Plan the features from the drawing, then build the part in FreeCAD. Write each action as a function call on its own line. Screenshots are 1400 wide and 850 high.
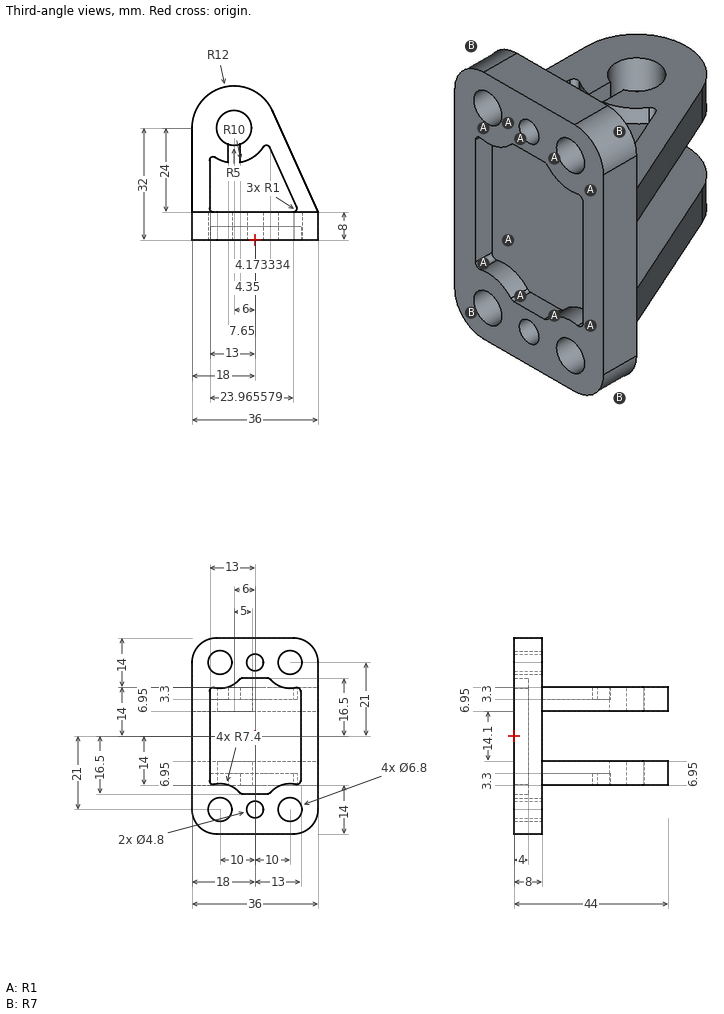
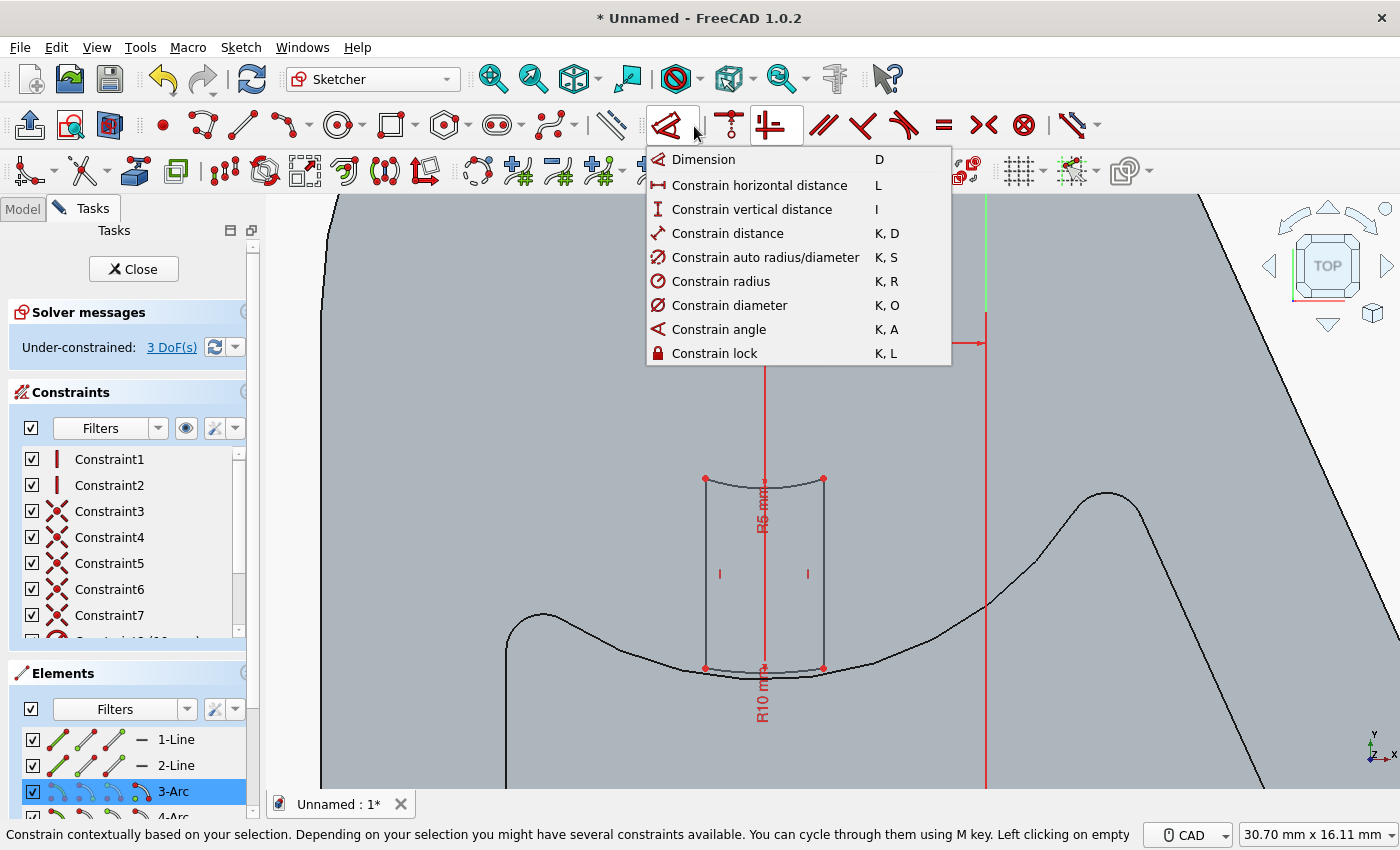
click(799, 209)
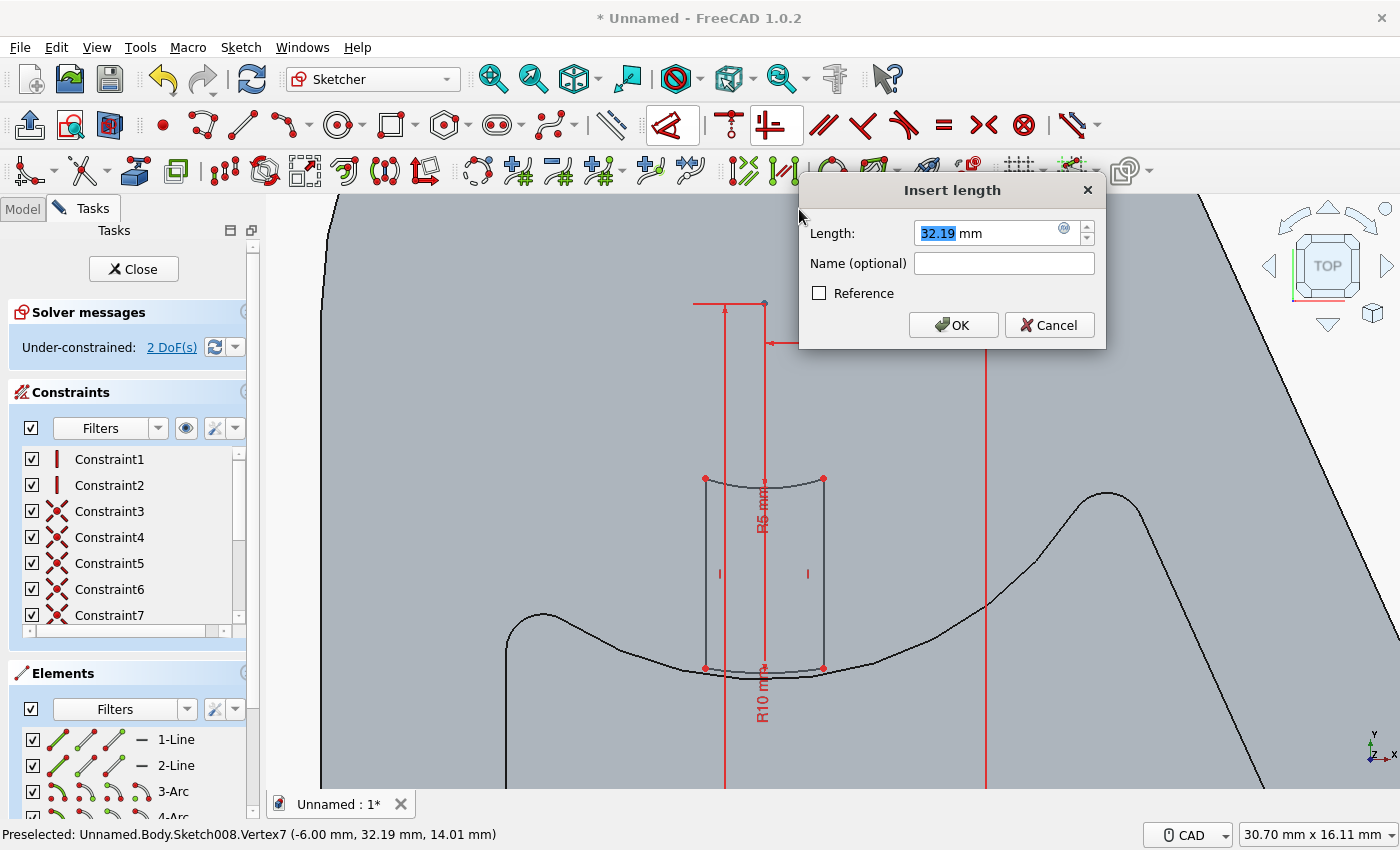
text(32)
key(Return)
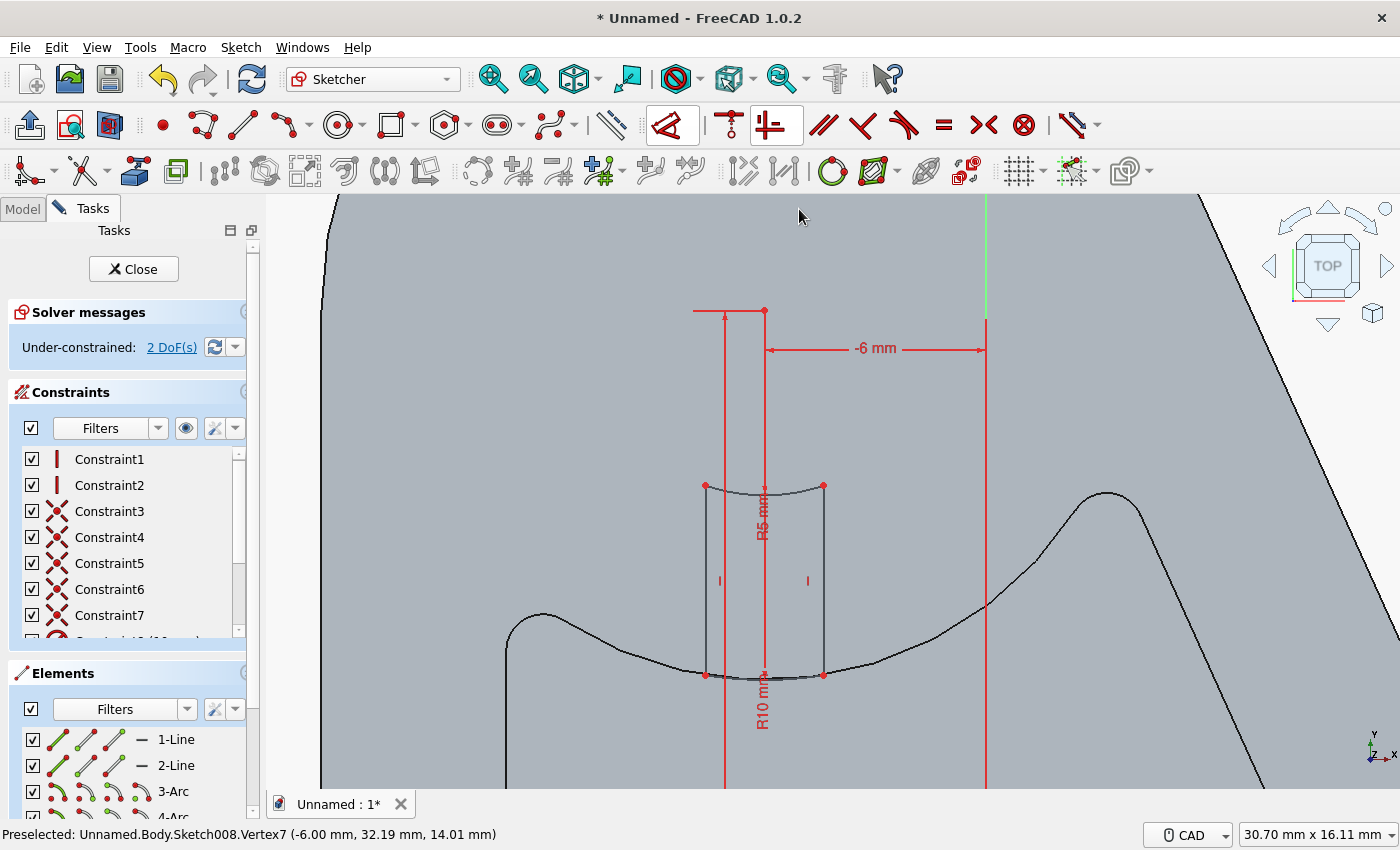
click(706, 486)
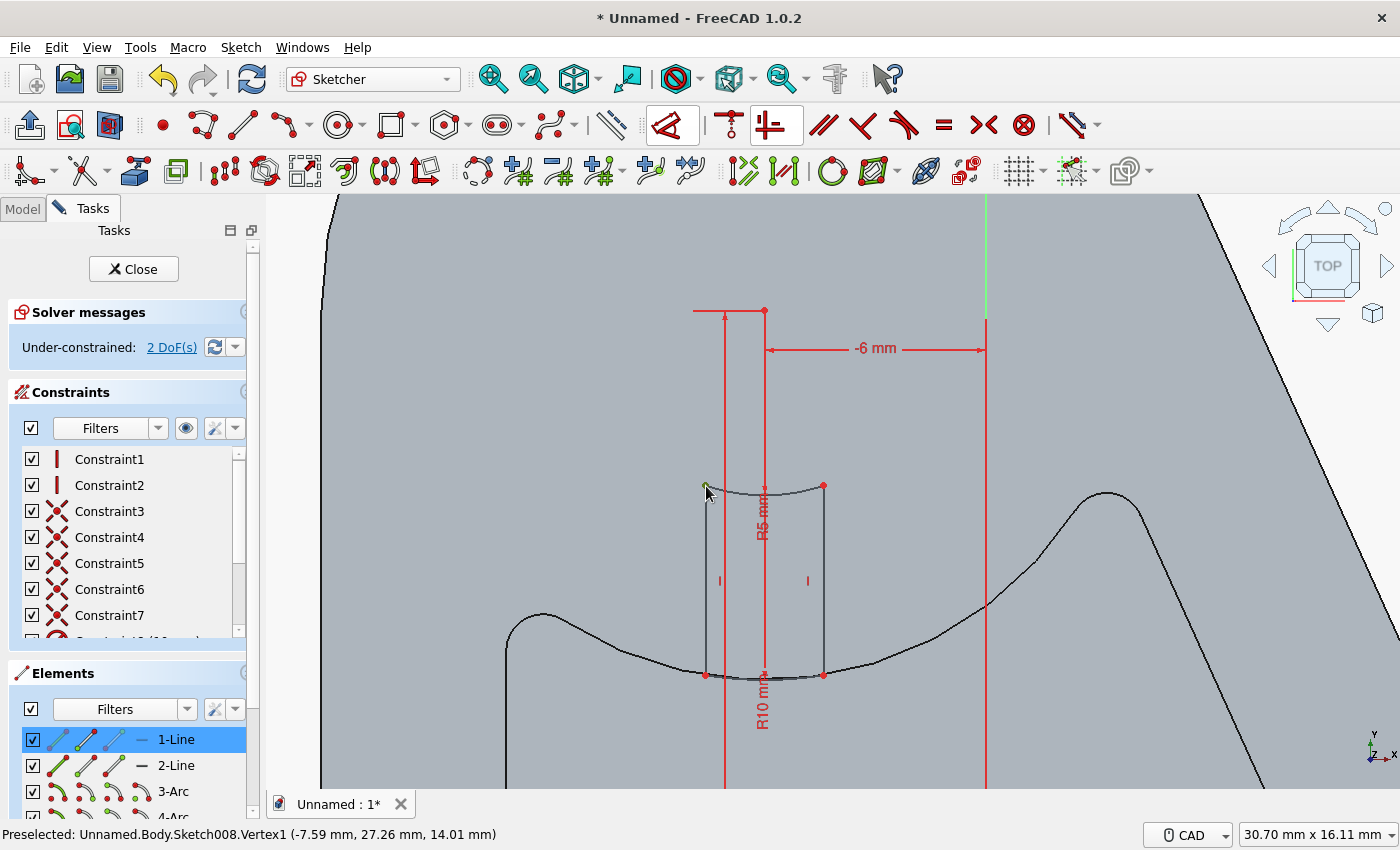
click(694, 126)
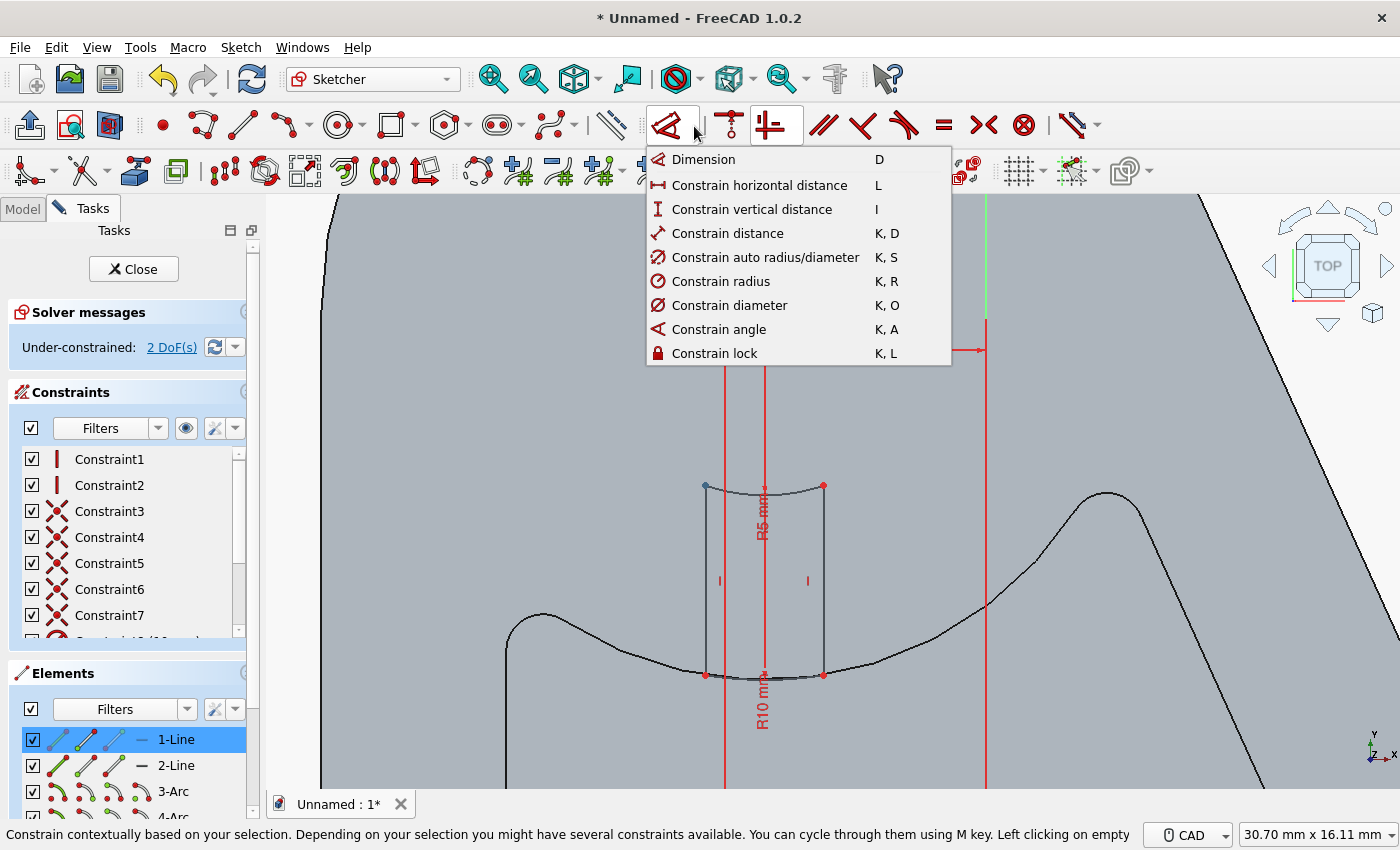
click(799, 185)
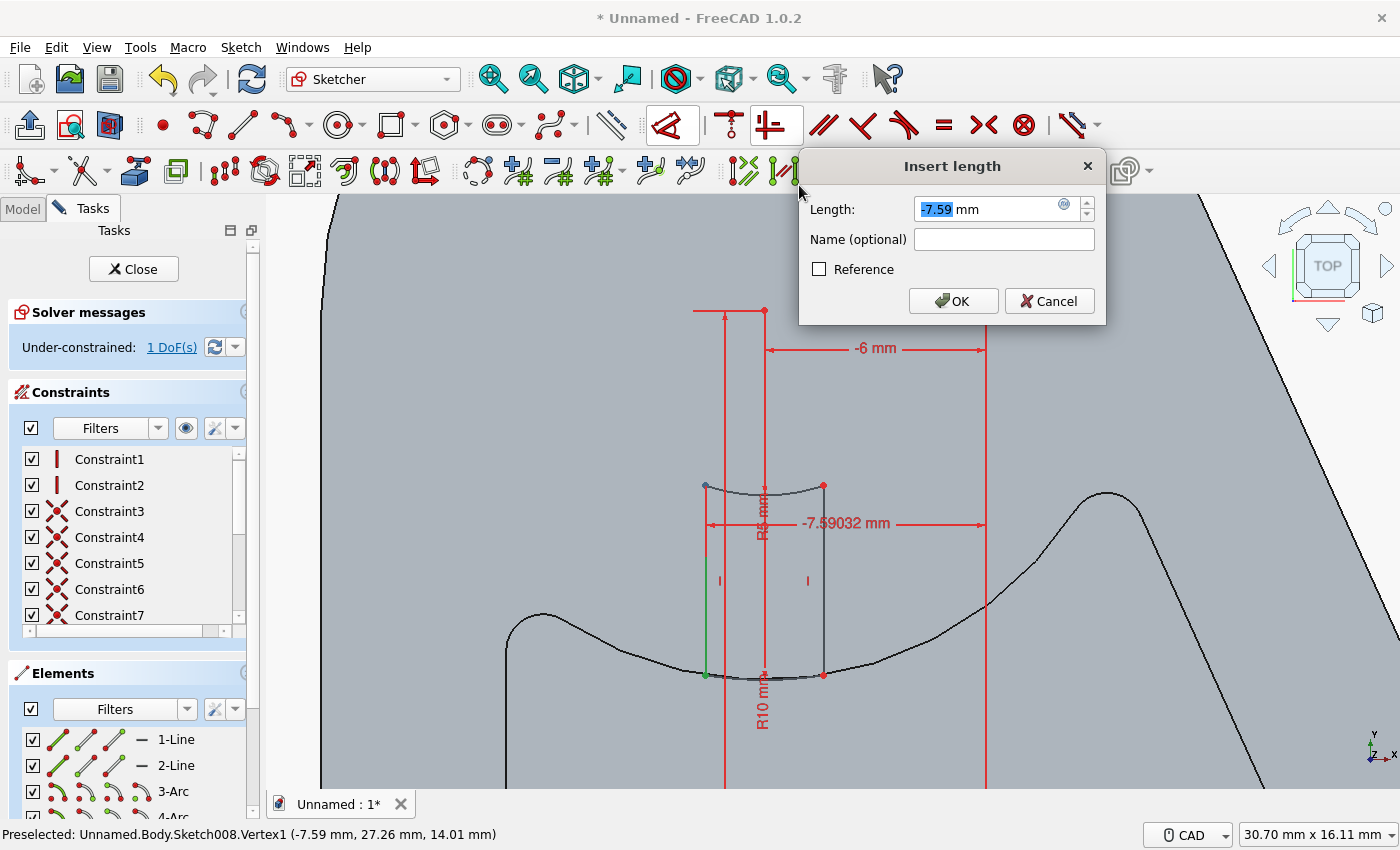
text(-7.65)
key(Return)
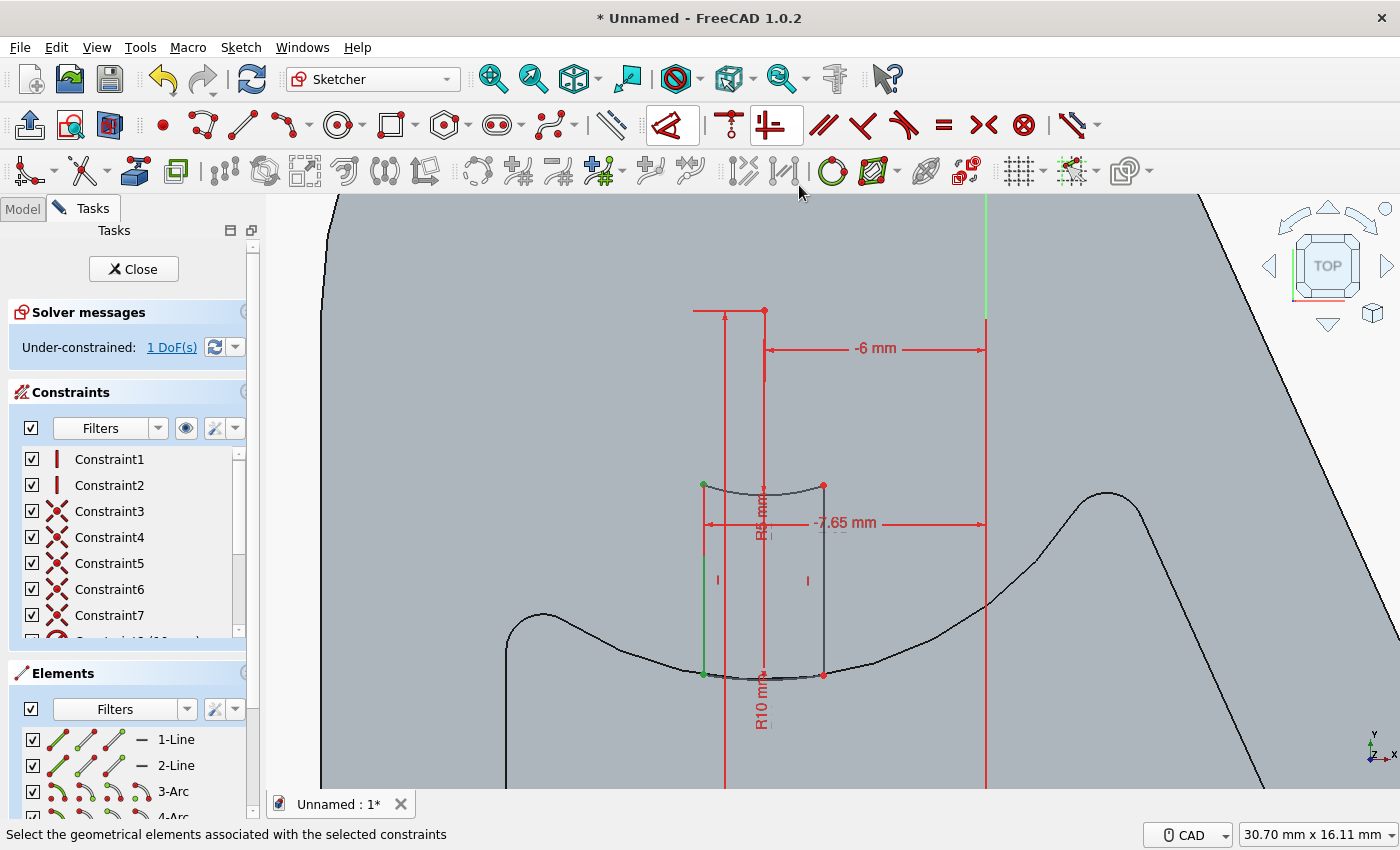
click(824, 675)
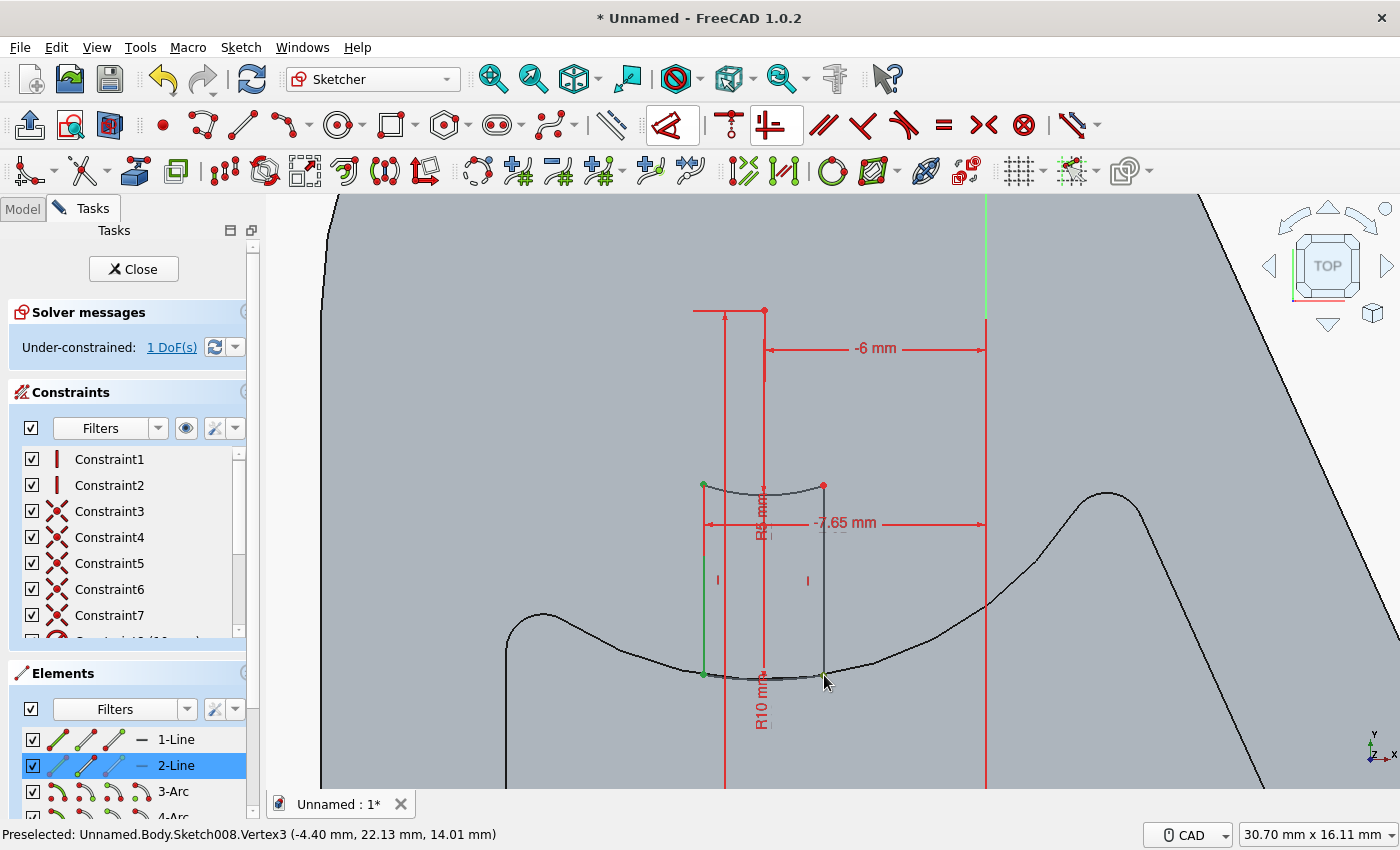
click(694, 126)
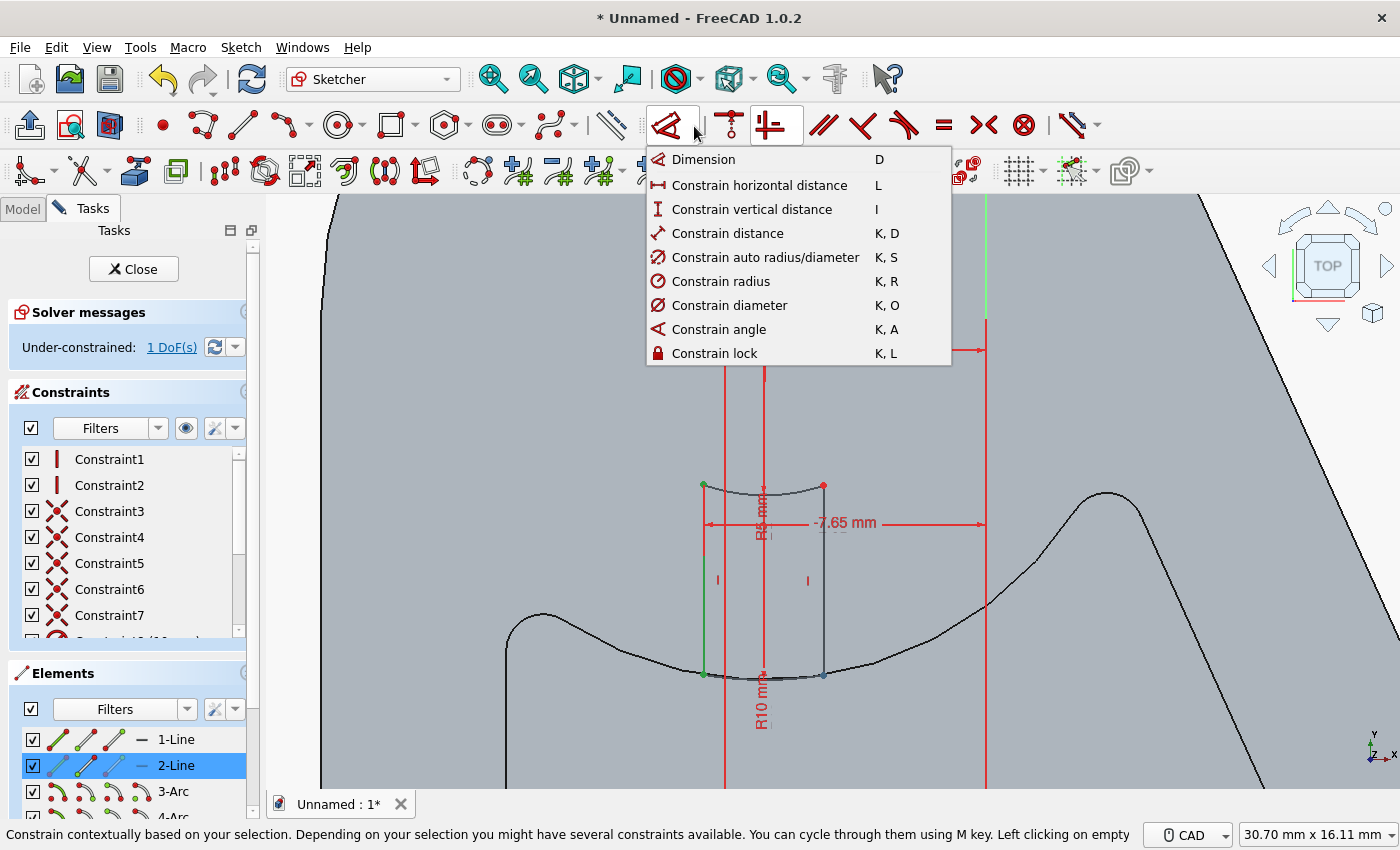
click(799, 185)